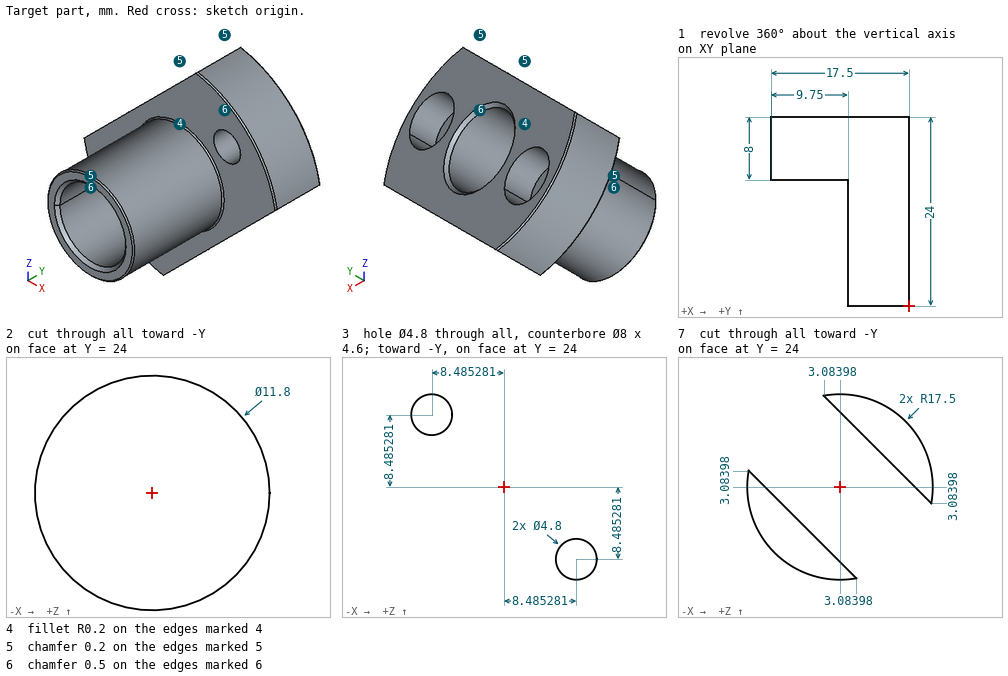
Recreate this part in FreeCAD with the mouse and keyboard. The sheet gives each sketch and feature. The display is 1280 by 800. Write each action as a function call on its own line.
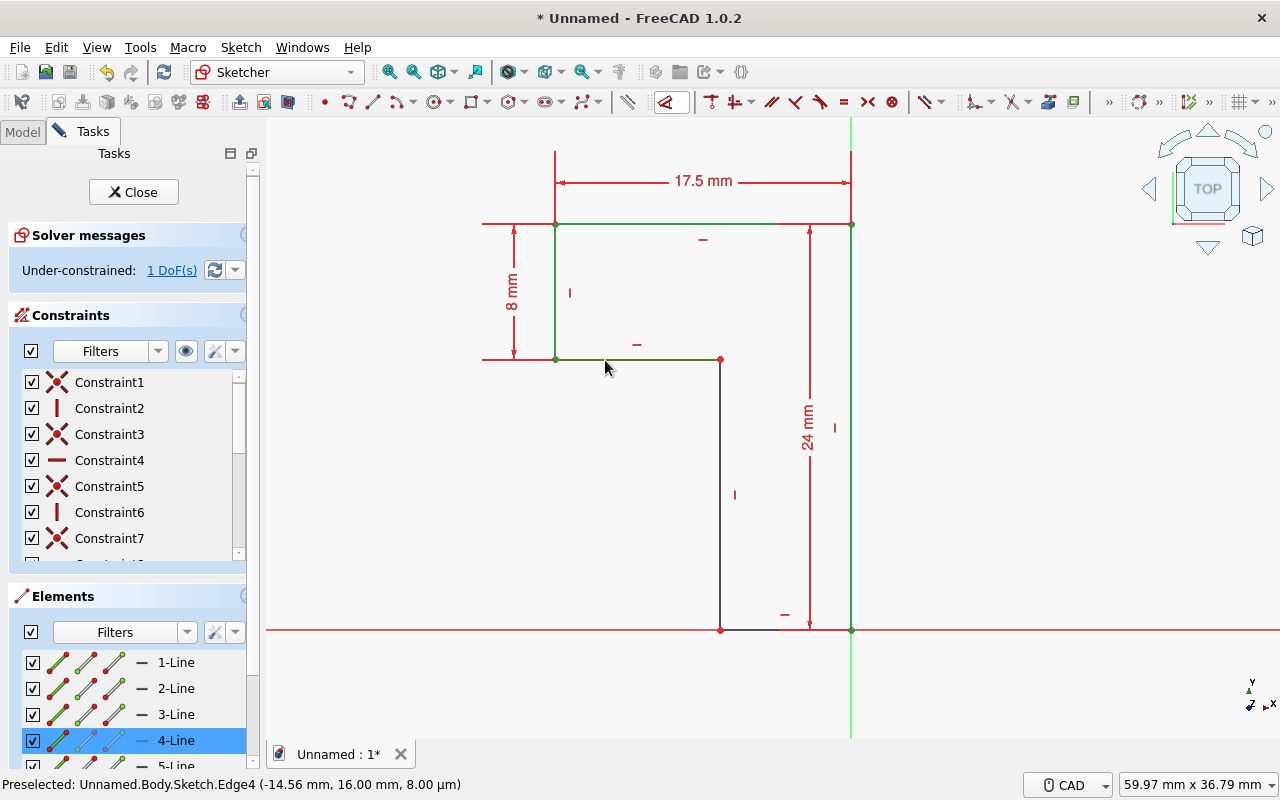
key(l)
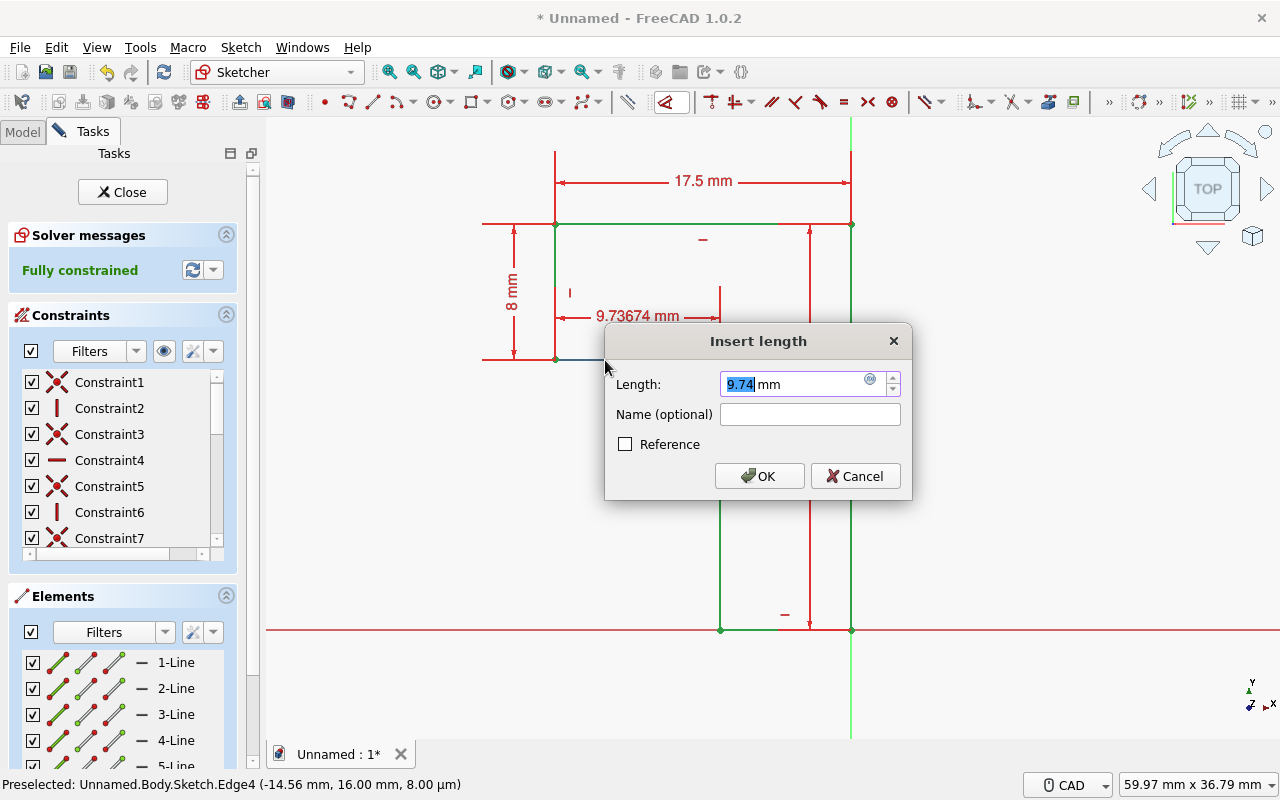
text(9.75)
key(Return)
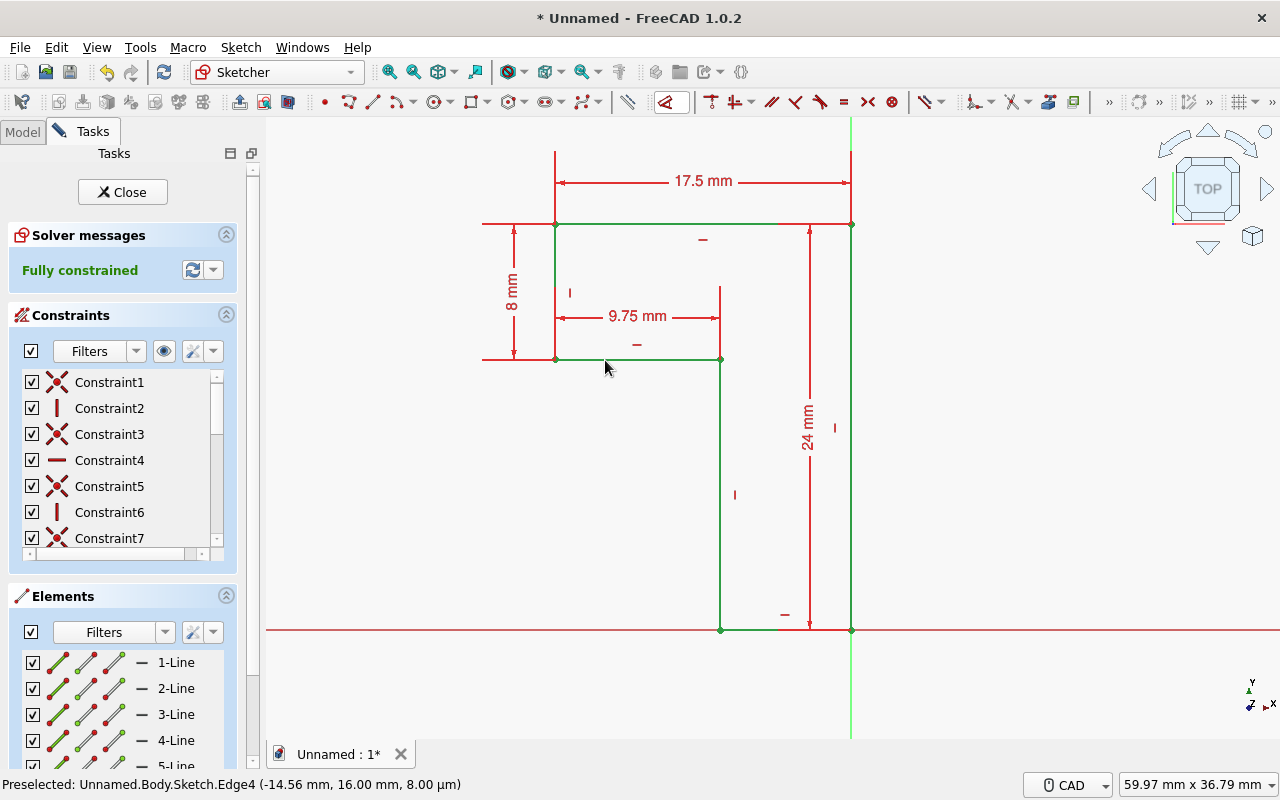
click(123, 192)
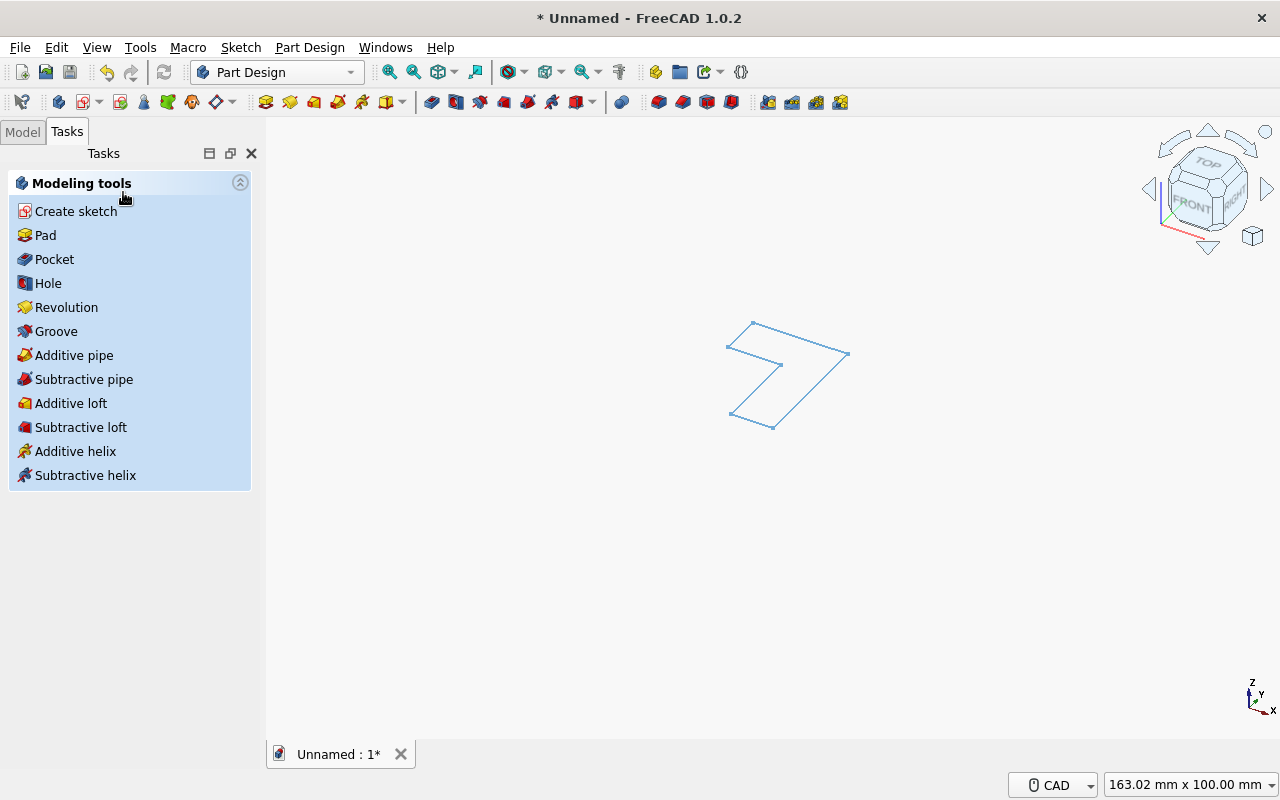
click(290, 102)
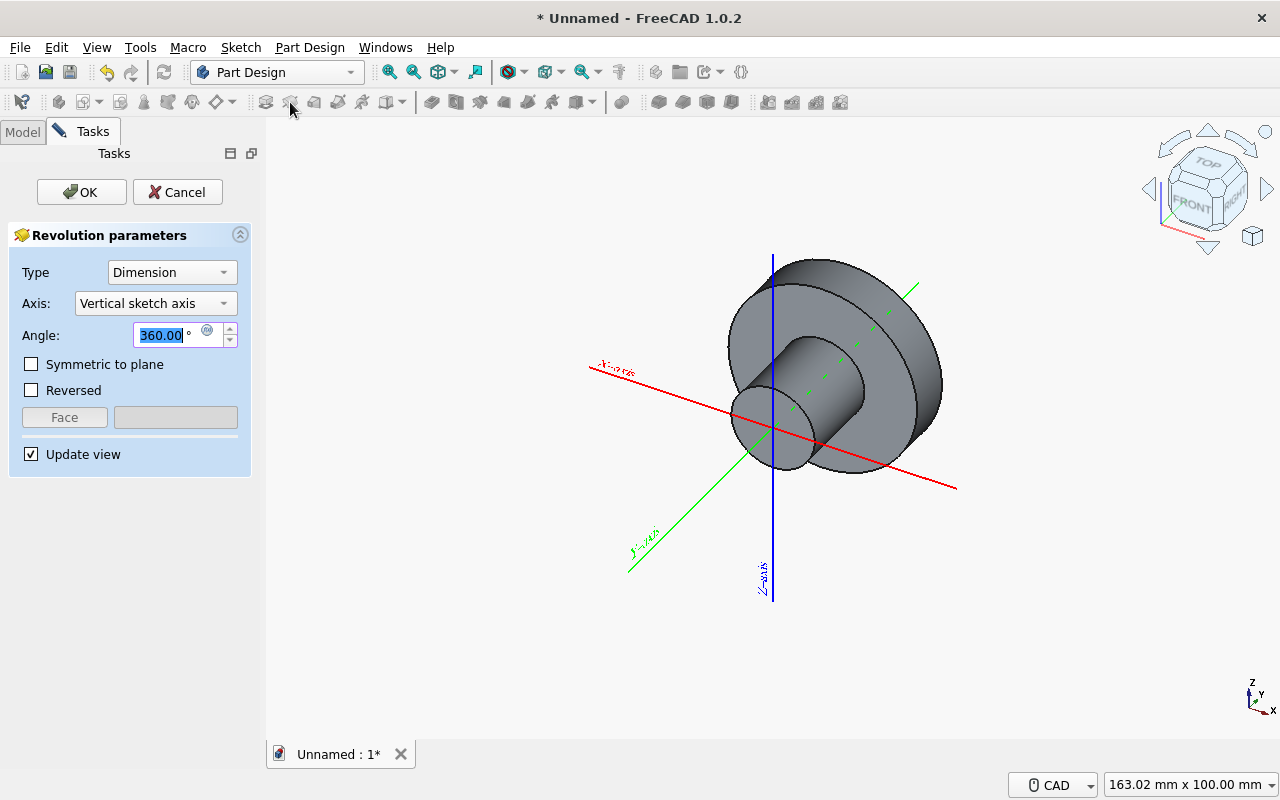
click(82, 192)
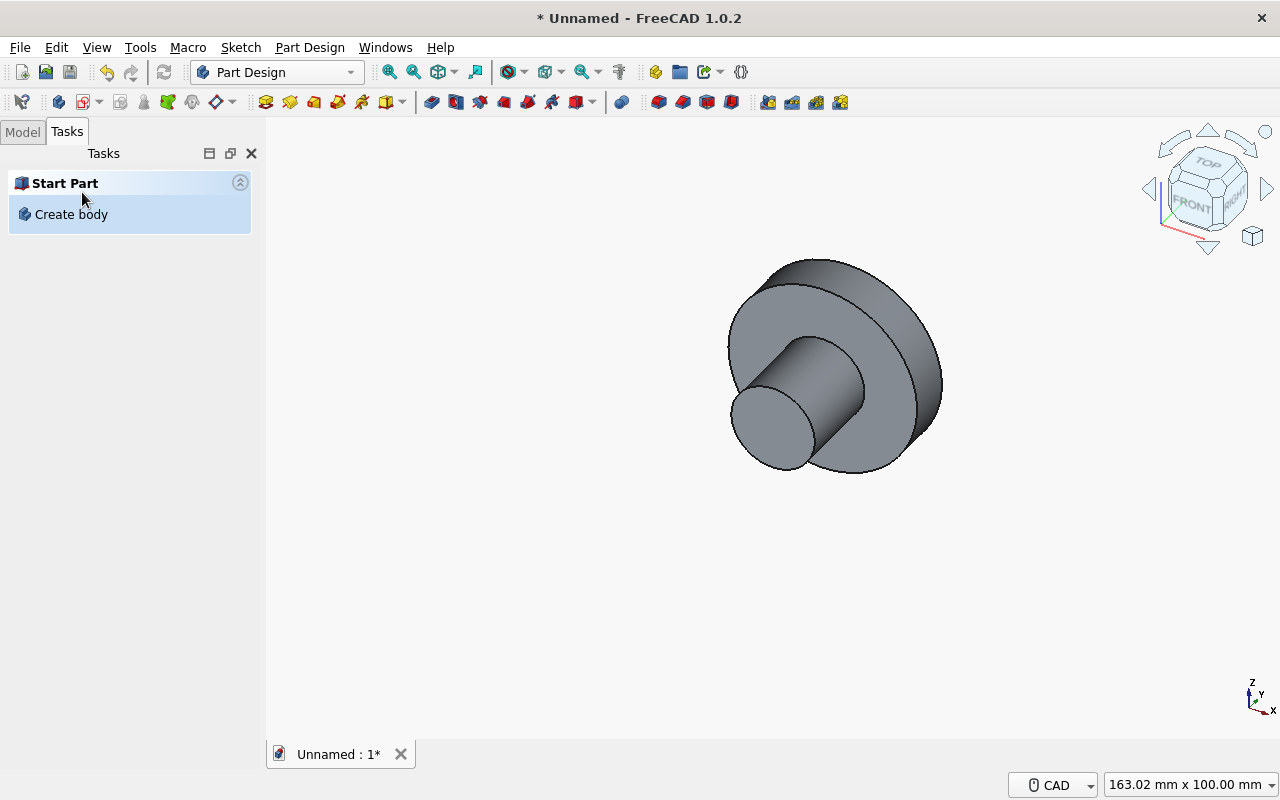
key(4)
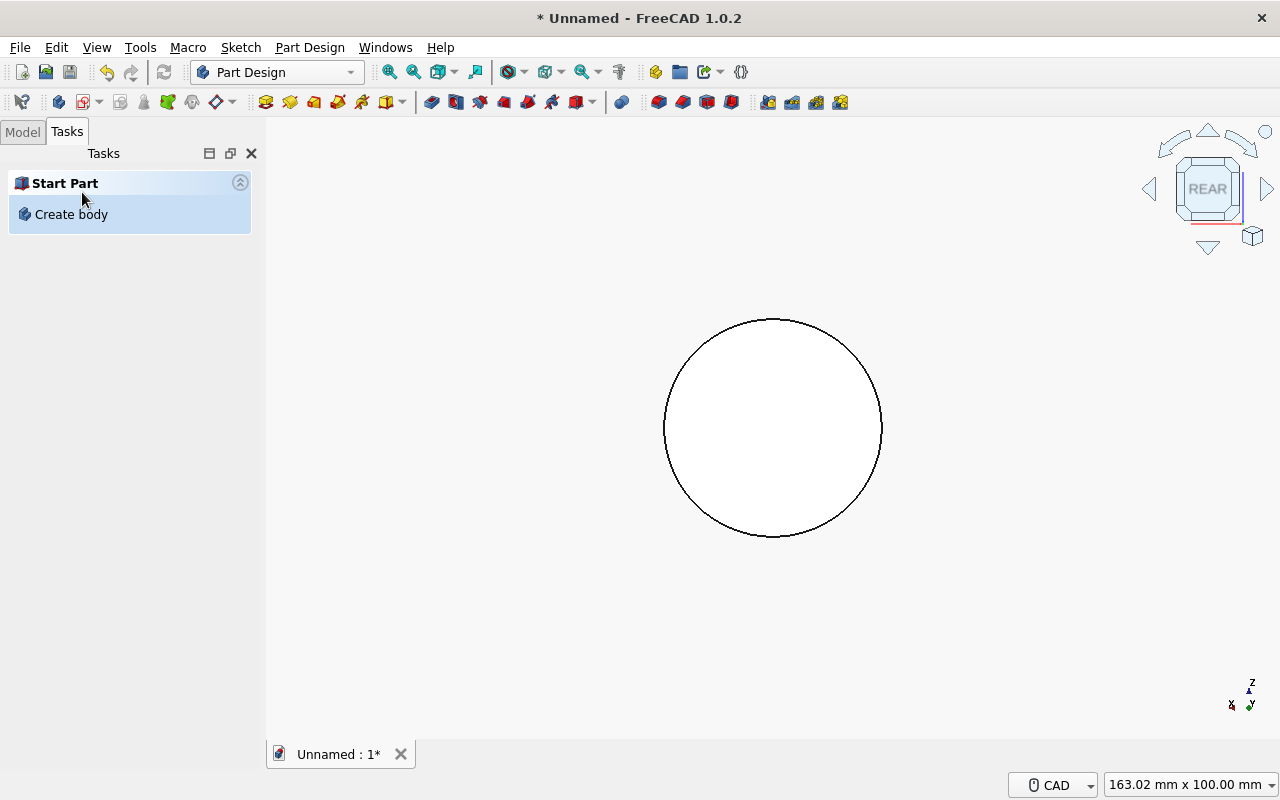
click(390, 72)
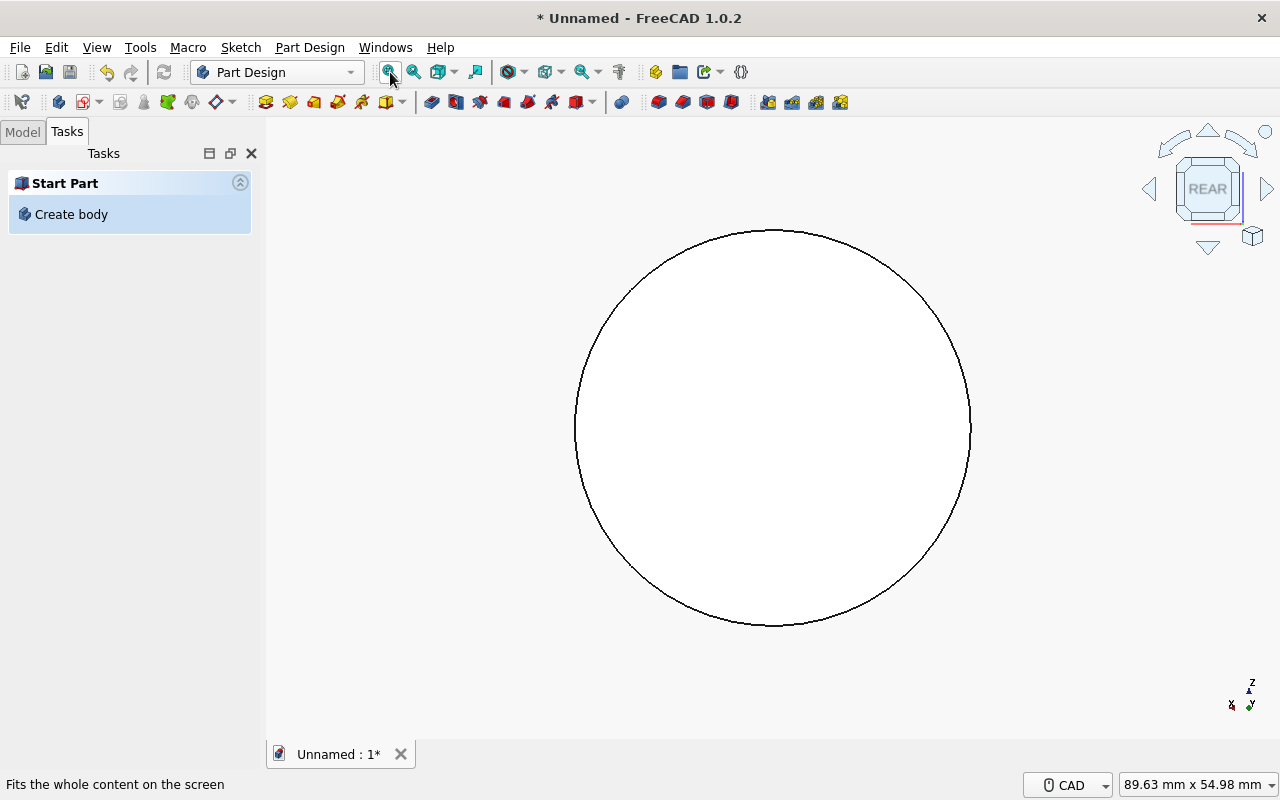
click(773, 427)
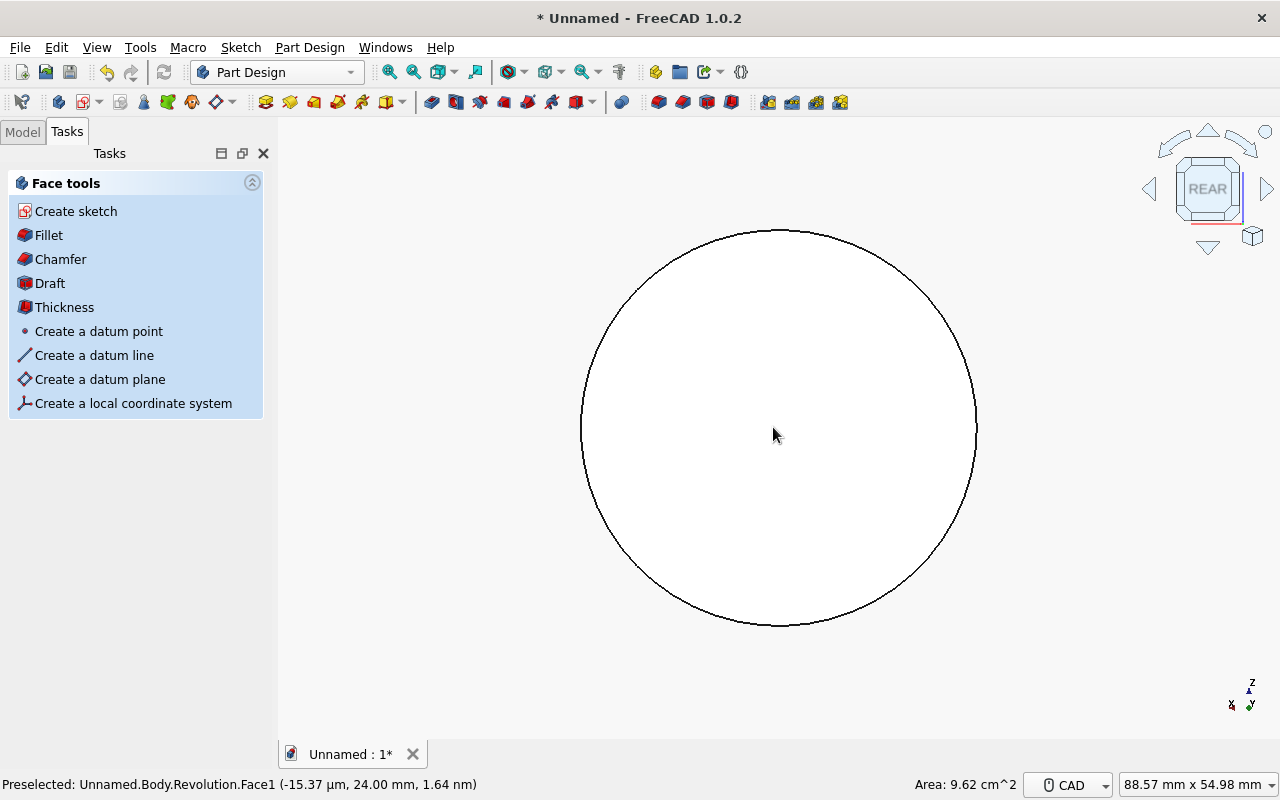
click(84, 102)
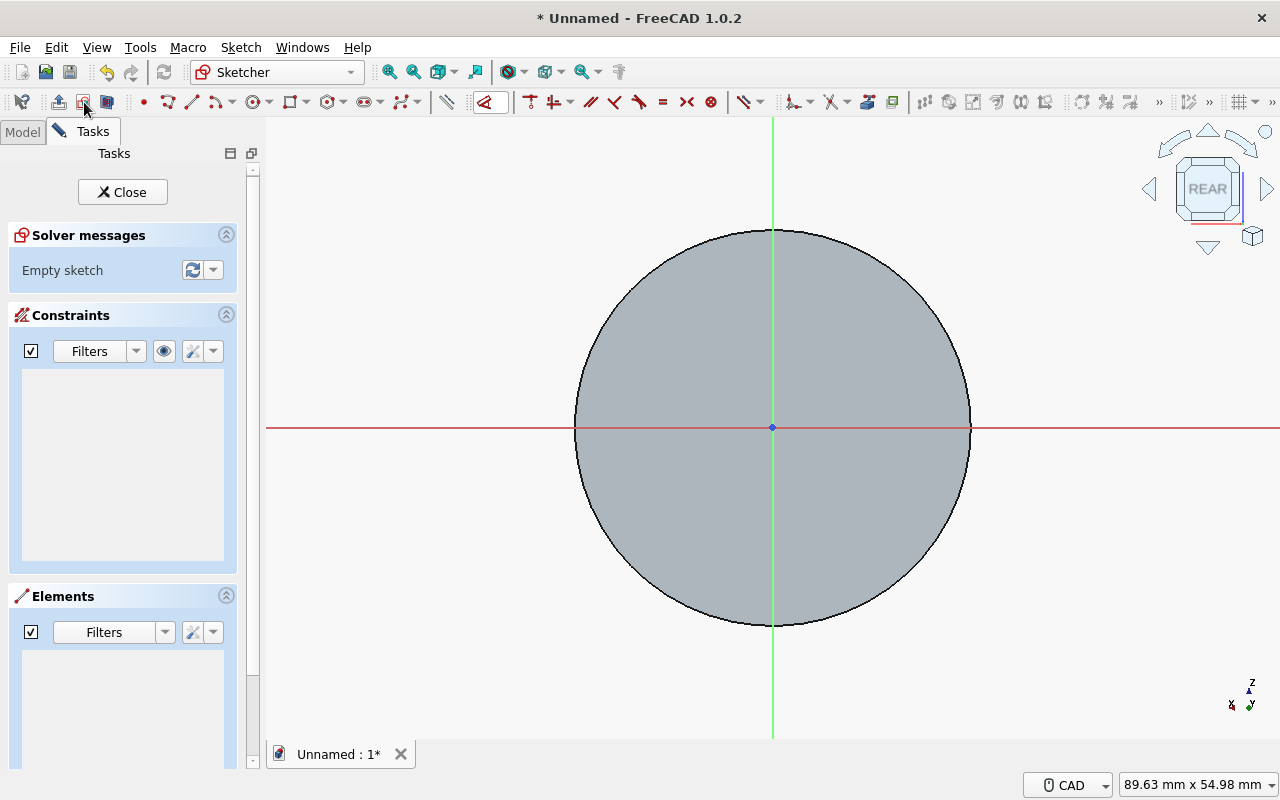
scroll(813, 428, up, 5)